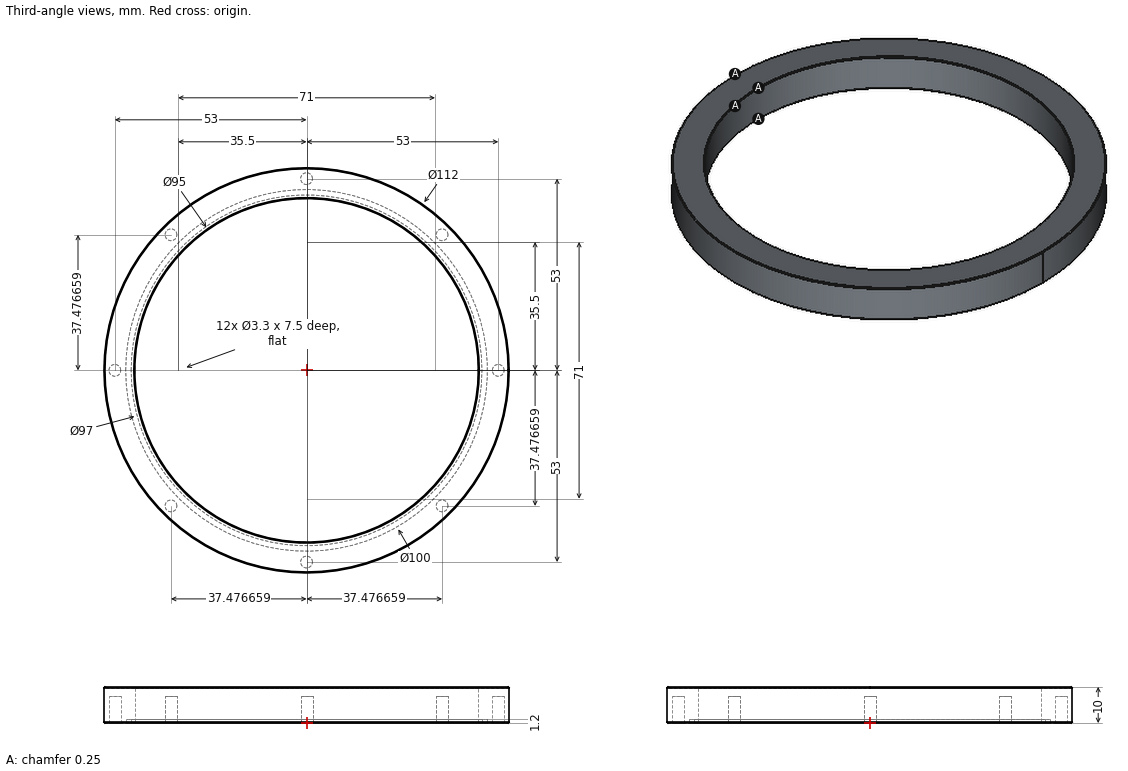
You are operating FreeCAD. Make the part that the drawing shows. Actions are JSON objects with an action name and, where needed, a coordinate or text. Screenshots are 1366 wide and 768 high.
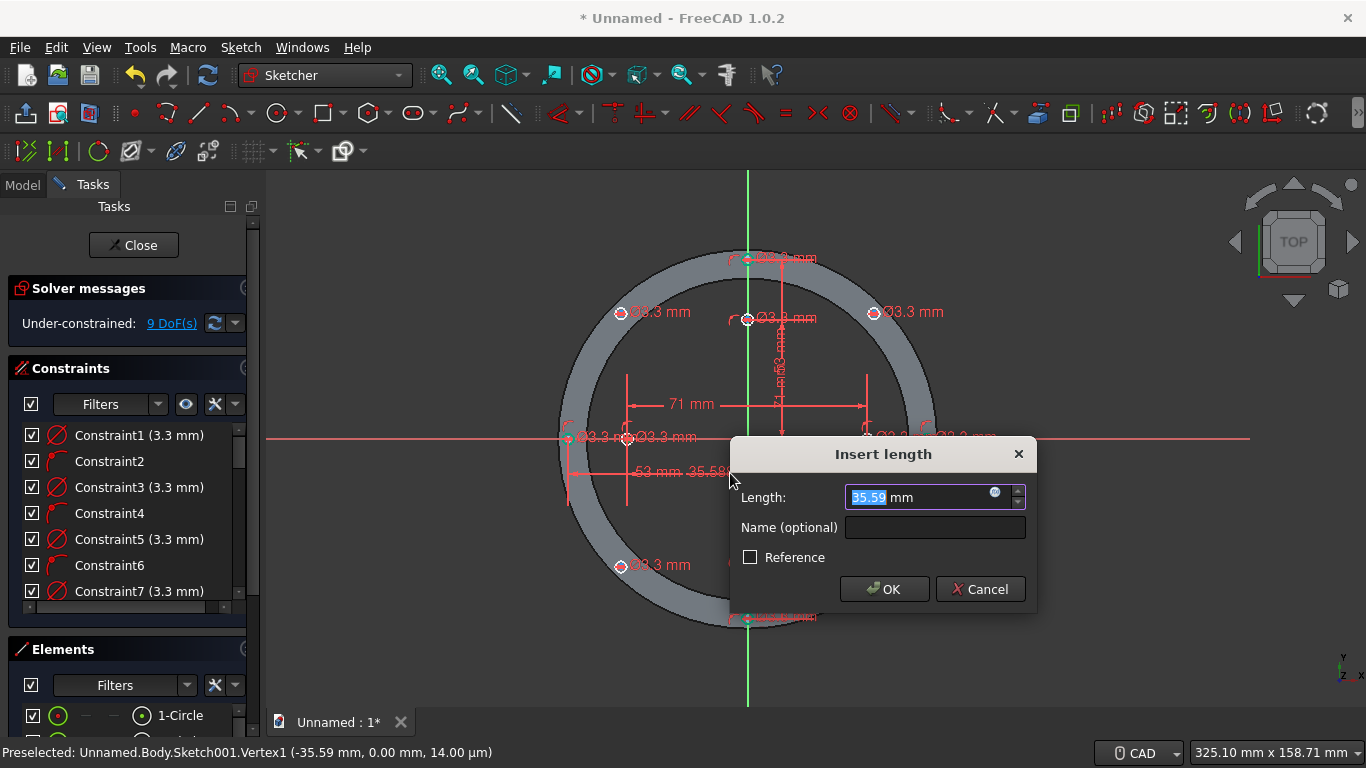
{"action": "type", "text": "35.5"}
{"action": "key", "text": "Return"}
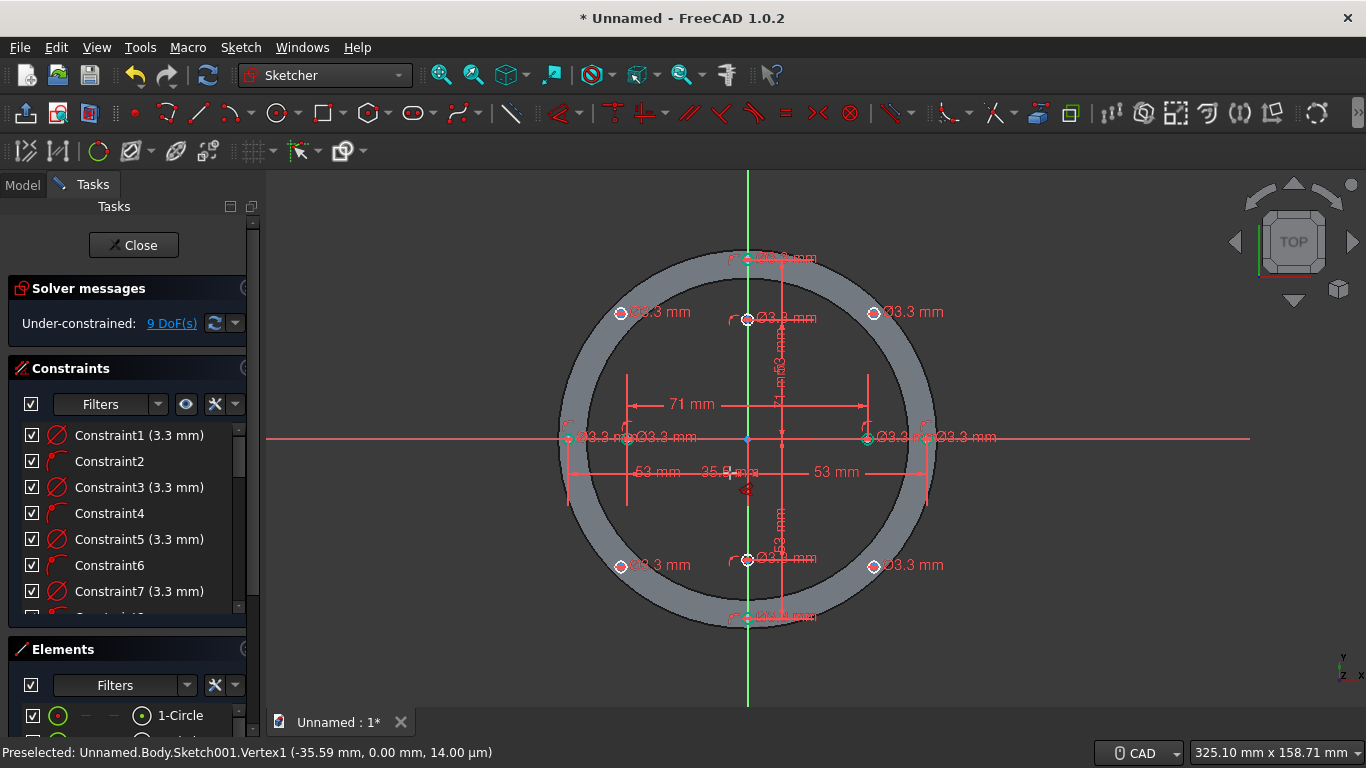
{"action": "left_click", "coordinate": [748, 320]}
{"action": "left_click", "coordinate": [782, 407]}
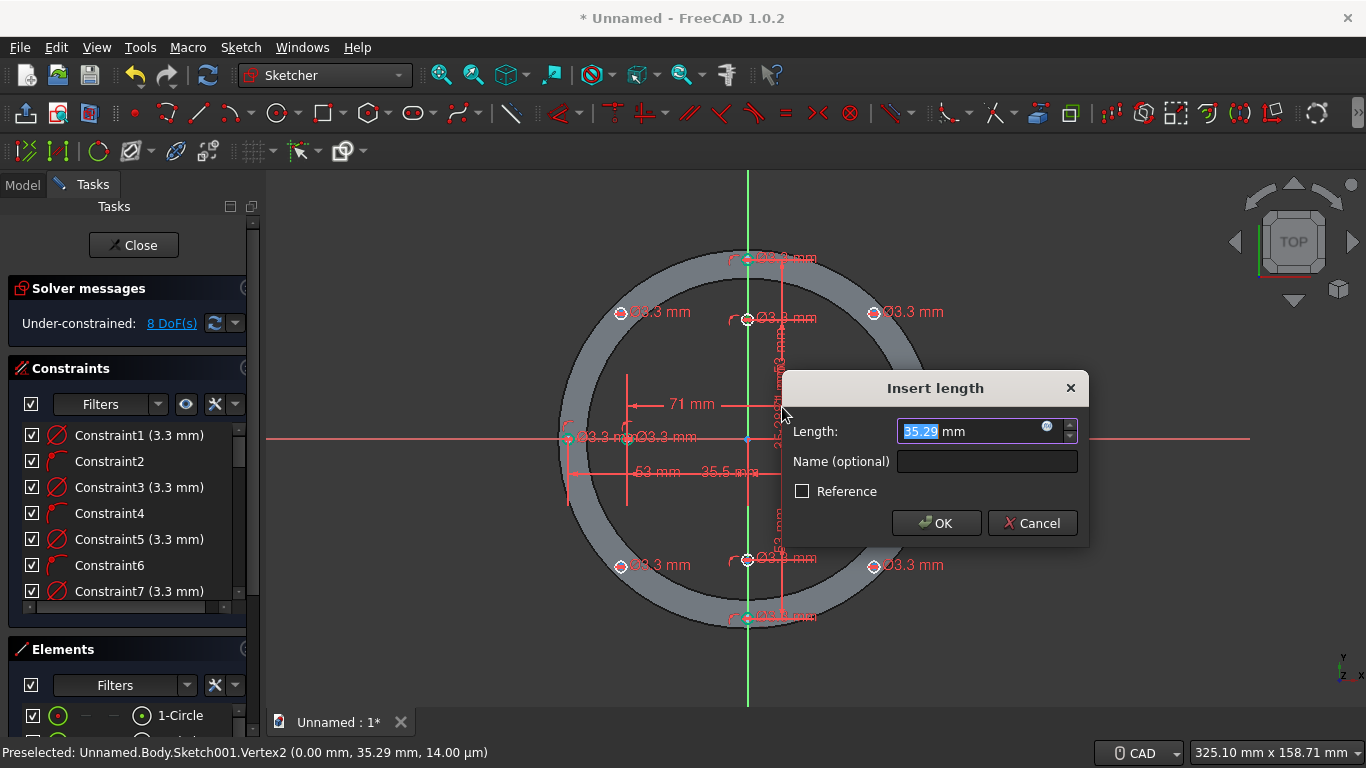
{"action": "type", "text": "35.5"}
{"action": "key", "text": "Return"}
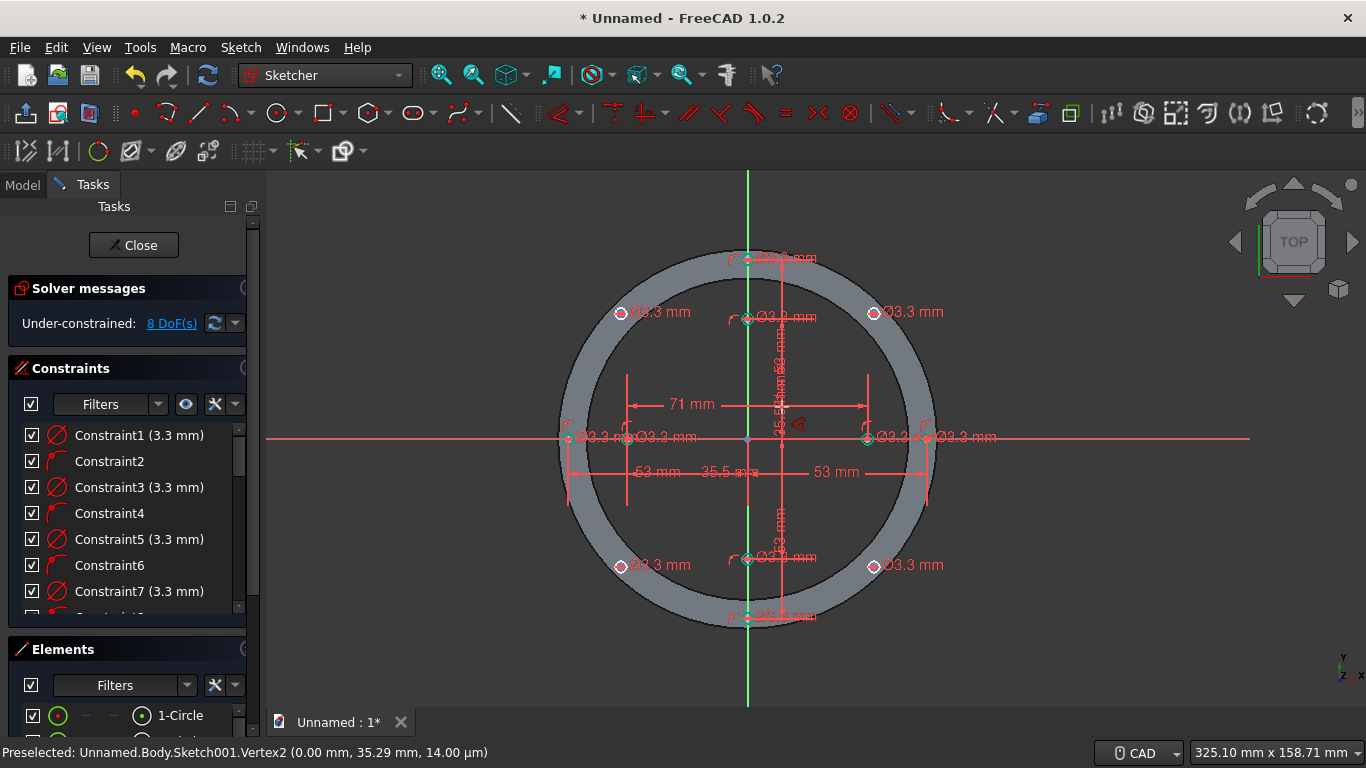
{"action": "left_click", "coordinate": [874, 567]}
{"action": "left_click", "coordinate": [811, 601]}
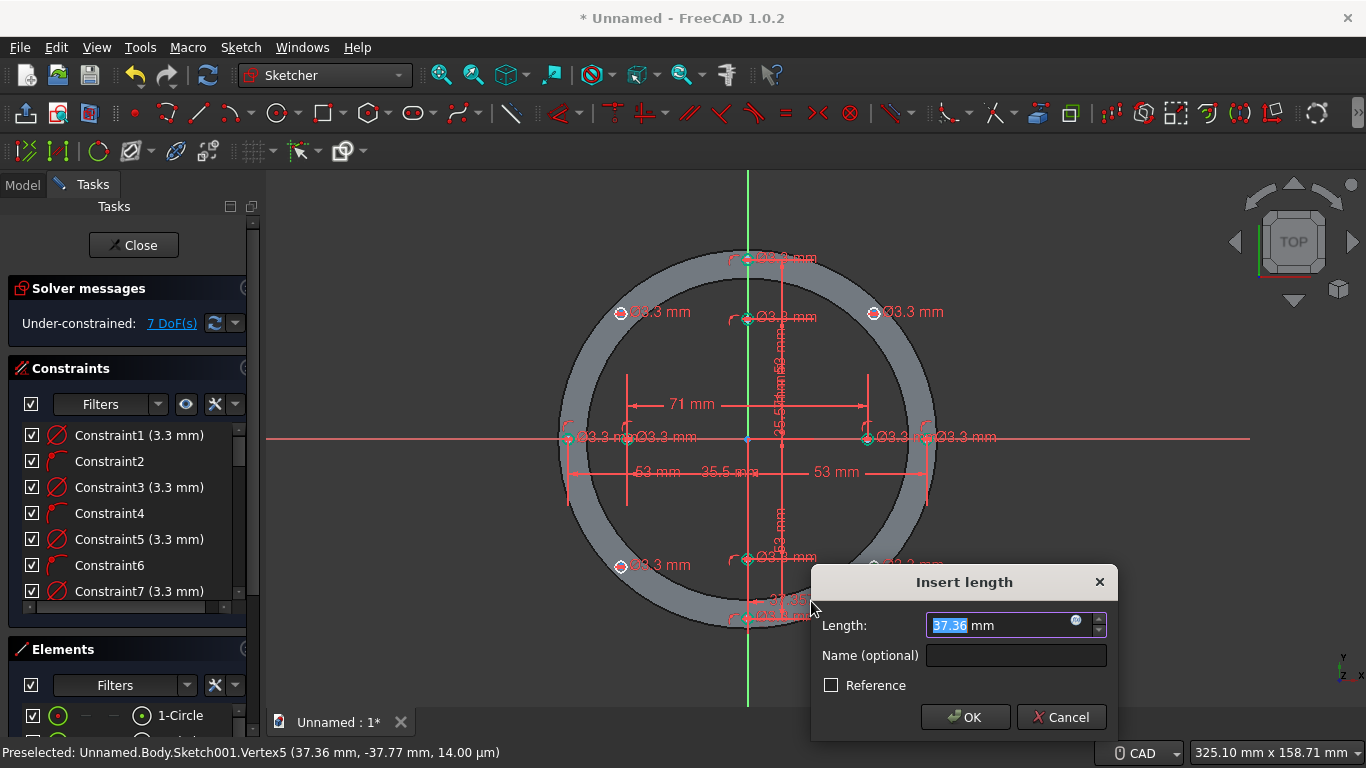
{"action": "type", "text": "37.476659"}
{"action": "key", "text": "Return"}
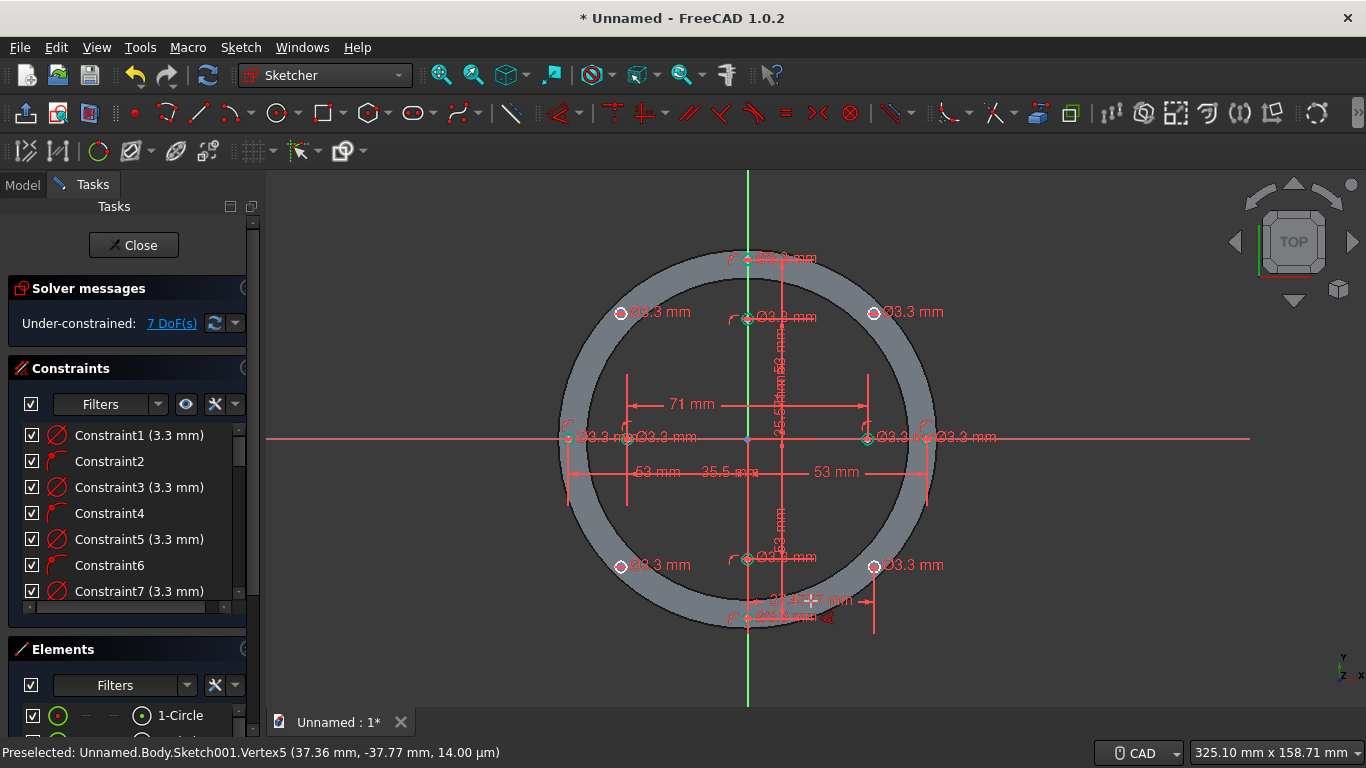
{"action": "left_click", "coordinate": [874, 567]}
{"action": "left_click", "coordinate": [908, 503]}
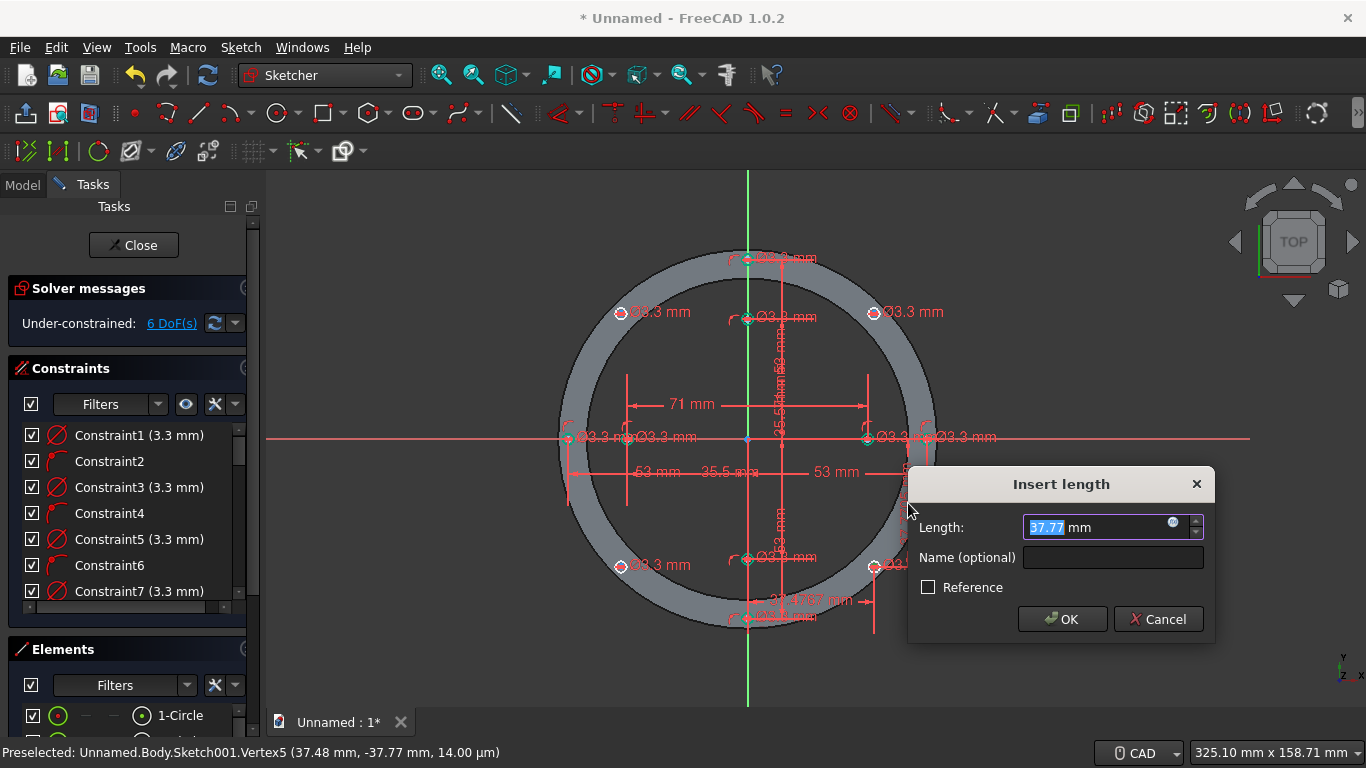
{"action": "type", "text": "37.476659"}
{"action": "key", "text": "Return"}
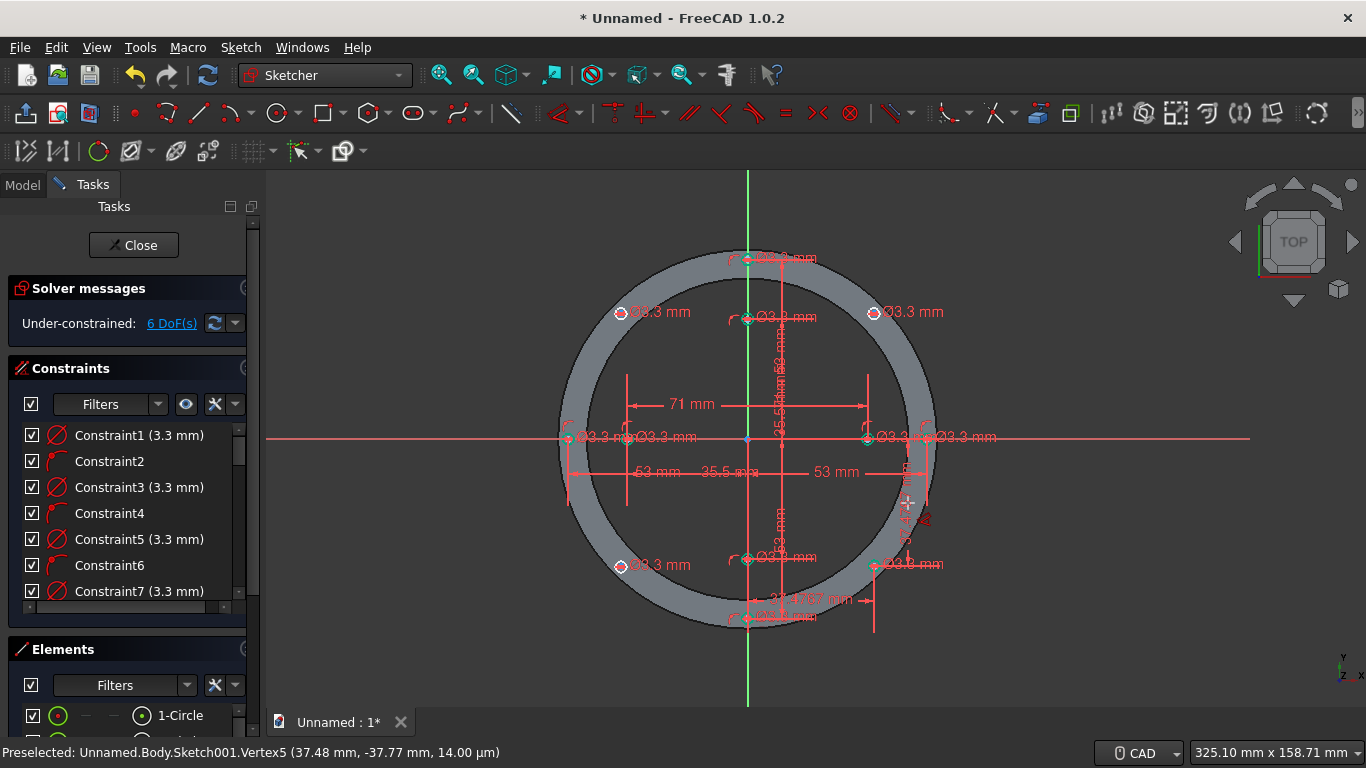
{"action": "left_click", "coordinate": [621, 567]}
{"action": "left_click", "coordinate": [684, 601]}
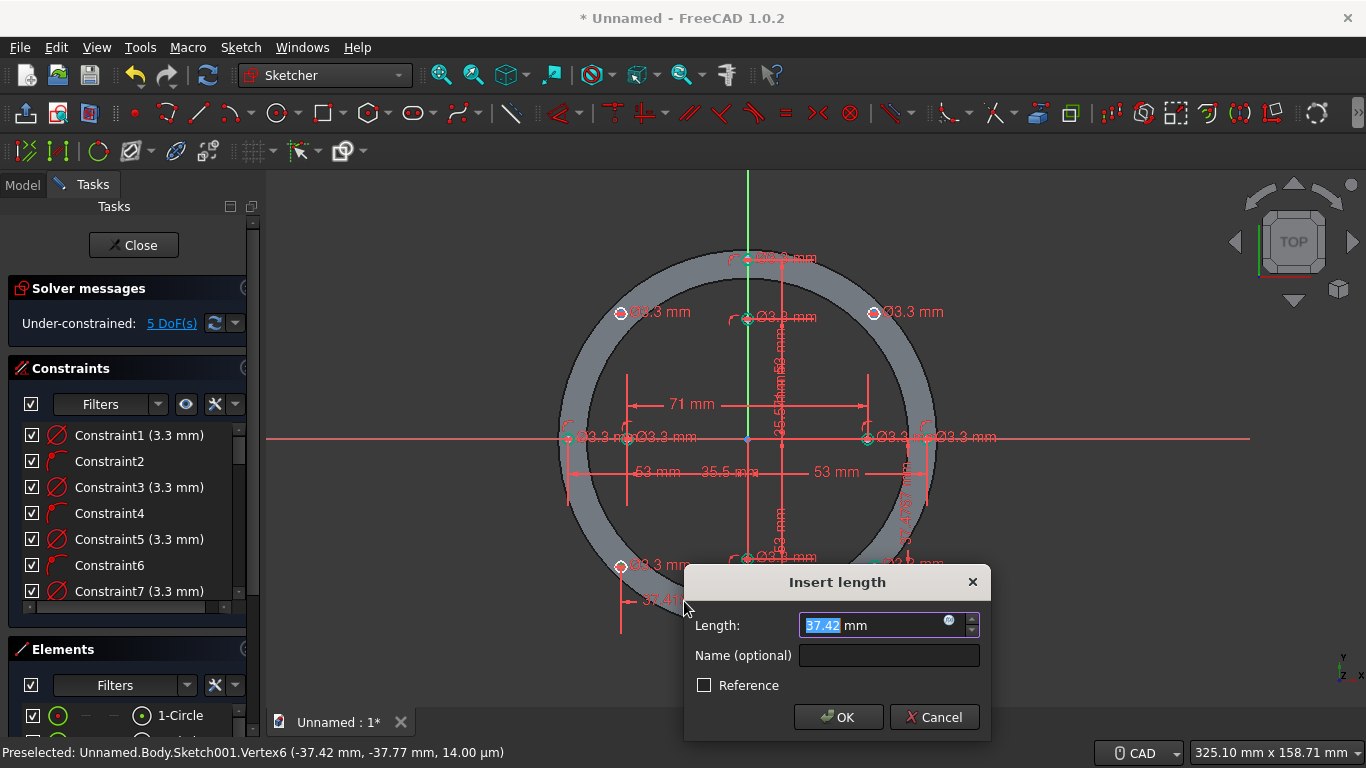
{"action": "type", "text": "37.476659"}
{"action": "key", "text": "Return"}